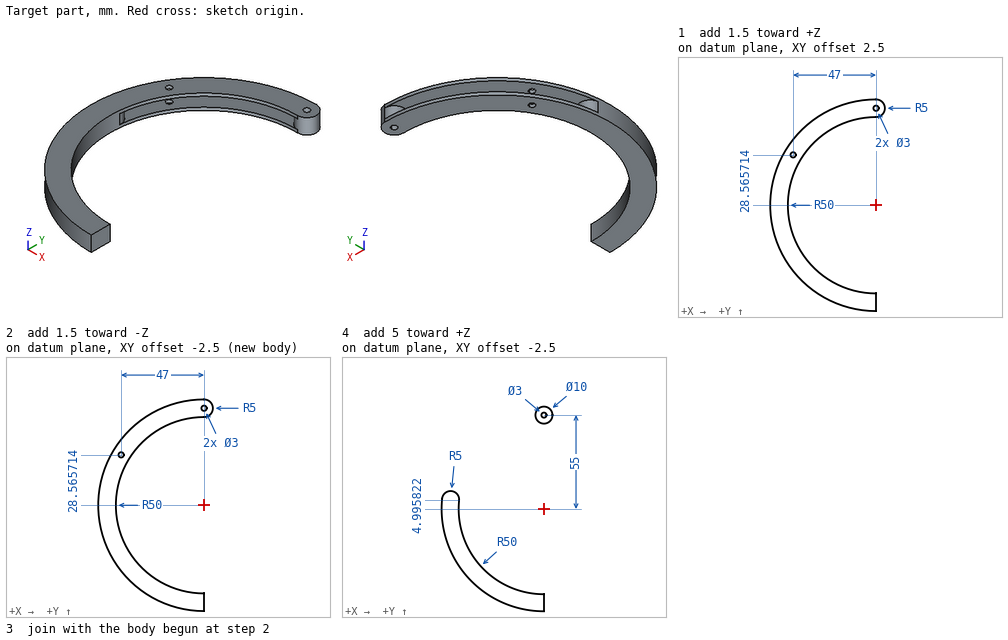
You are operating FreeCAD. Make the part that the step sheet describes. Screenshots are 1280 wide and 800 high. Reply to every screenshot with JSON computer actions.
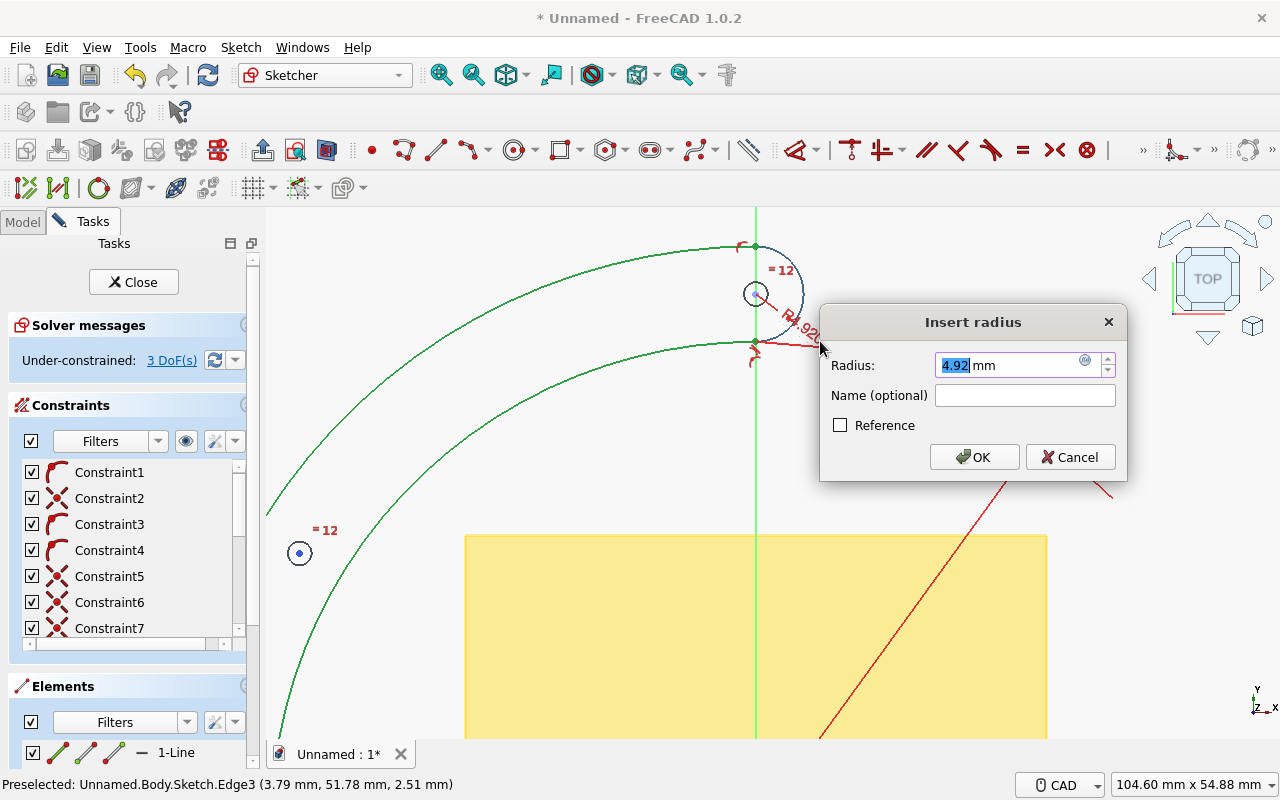
{"action": "type", "text": "5"}
{"action": "key", "text": "Return"}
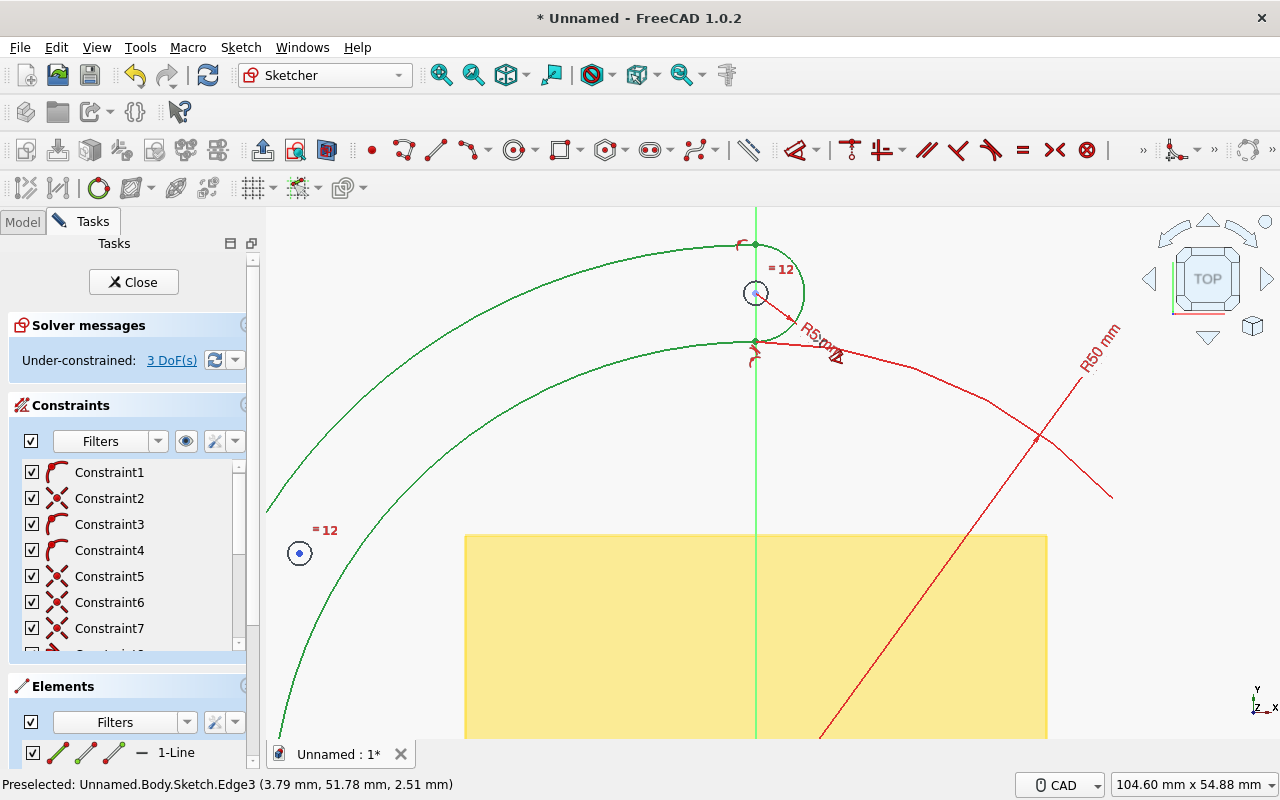
{"action": "scroll", "coordinate": [308, 545], "scroll_direction": "up", "scroll_amount": 2}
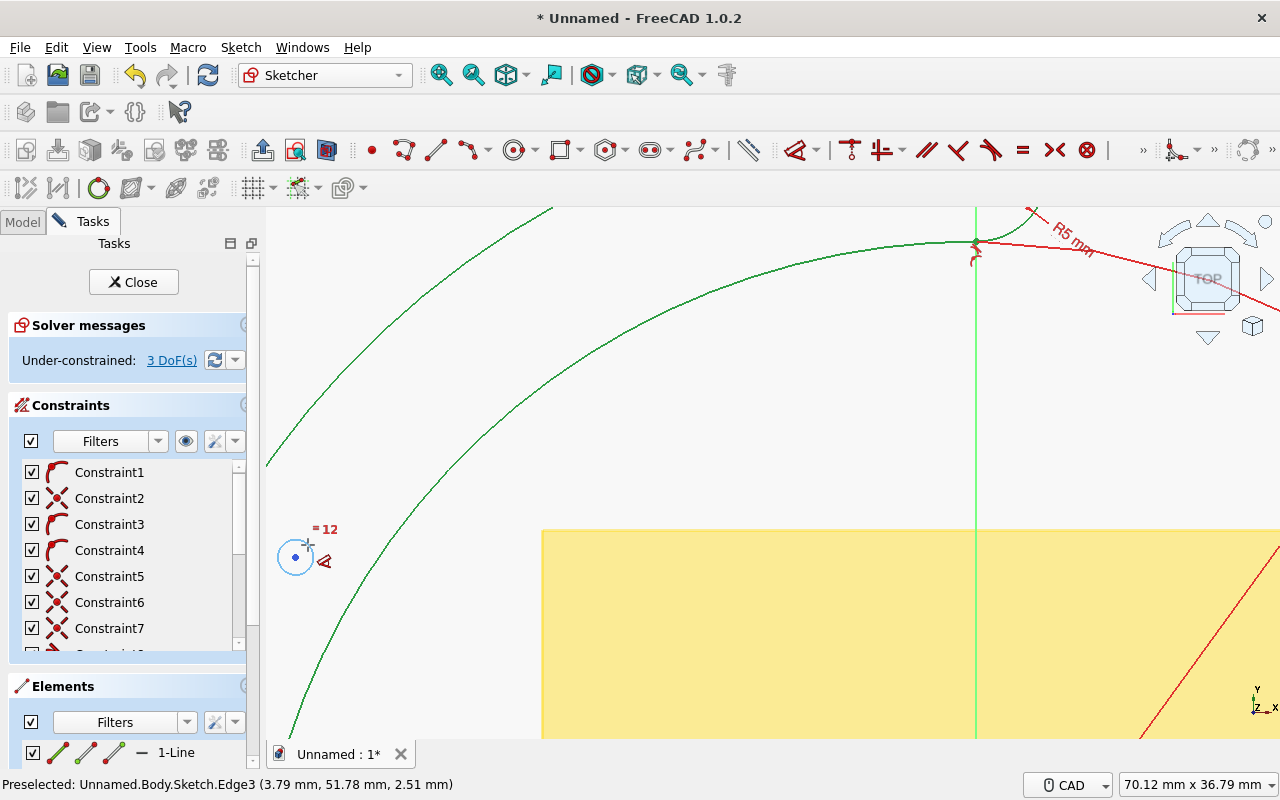
{"action": "left_click", "coordinate": [308, 545]}
{"action": "left_click", "coordinate": [331, 522]}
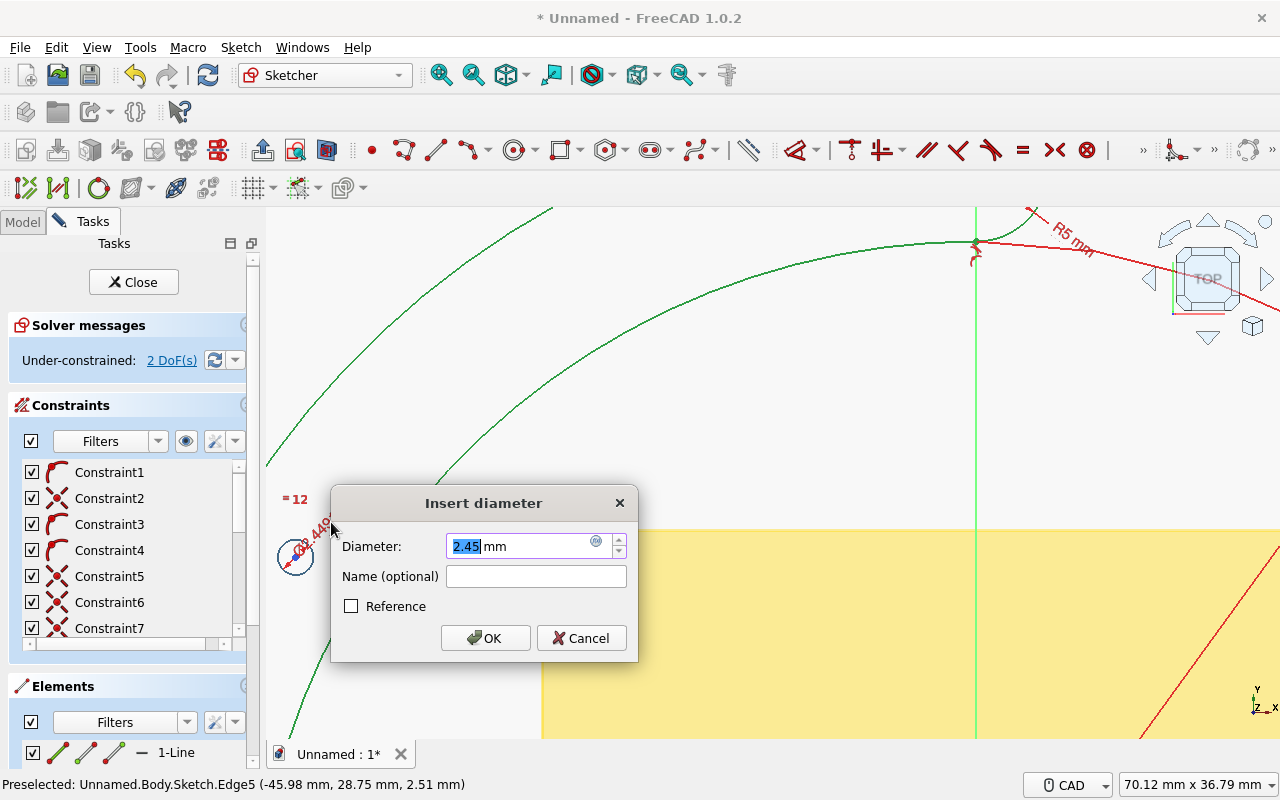
{"action": "type", "text": "3"}
{"action": "key", "text": "Return"}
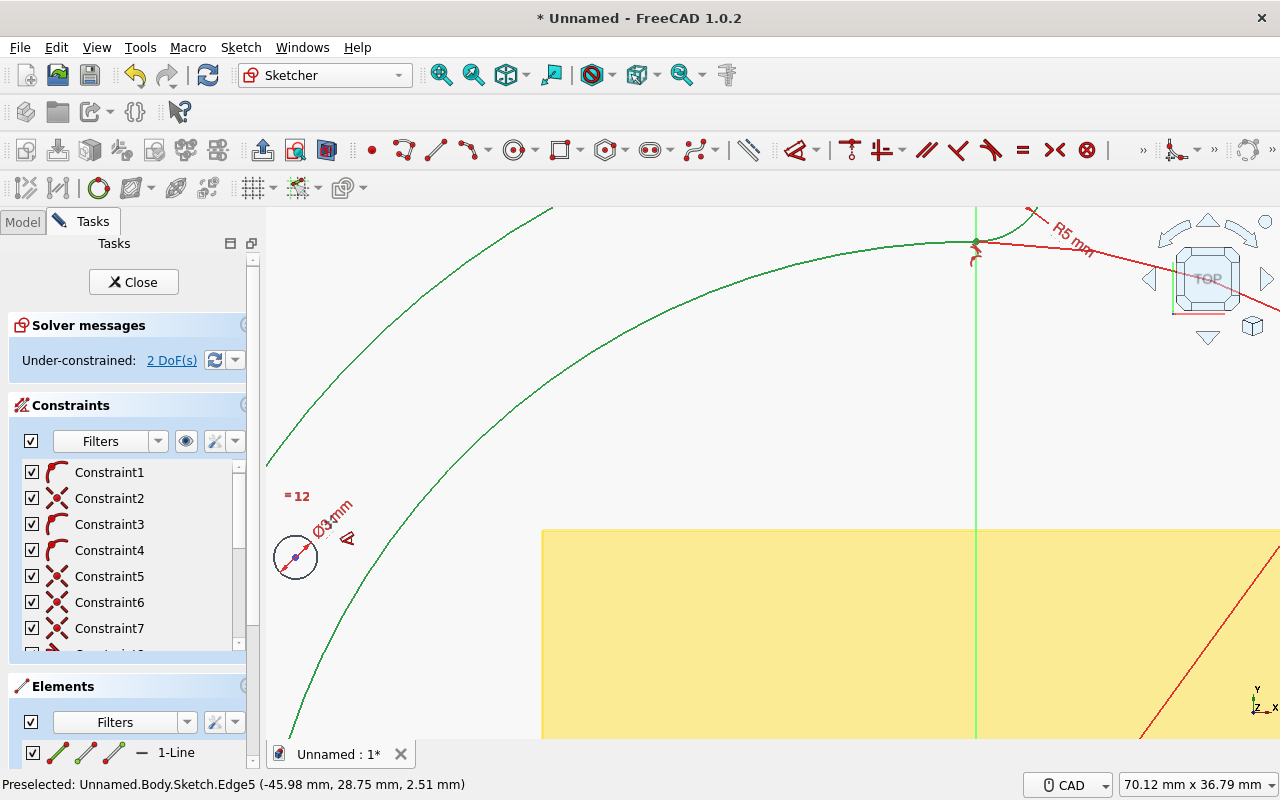
{"action": "scroll", "coordinate": [736, 349], "scroll_direction": "down", "scroll_amount": 8}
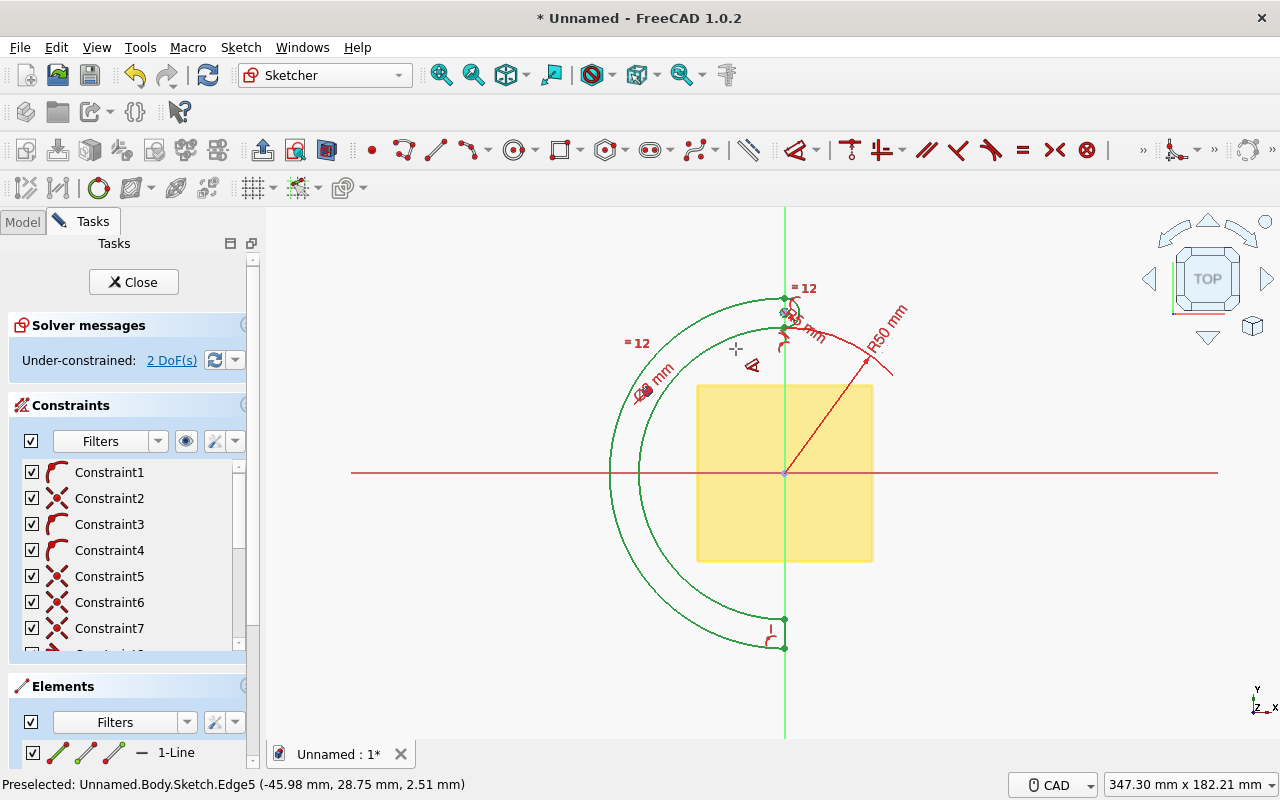
{"action": "left_click", "coordinate": [647, 391]}
{"action": "left_click", "coordinate": [748, 357]}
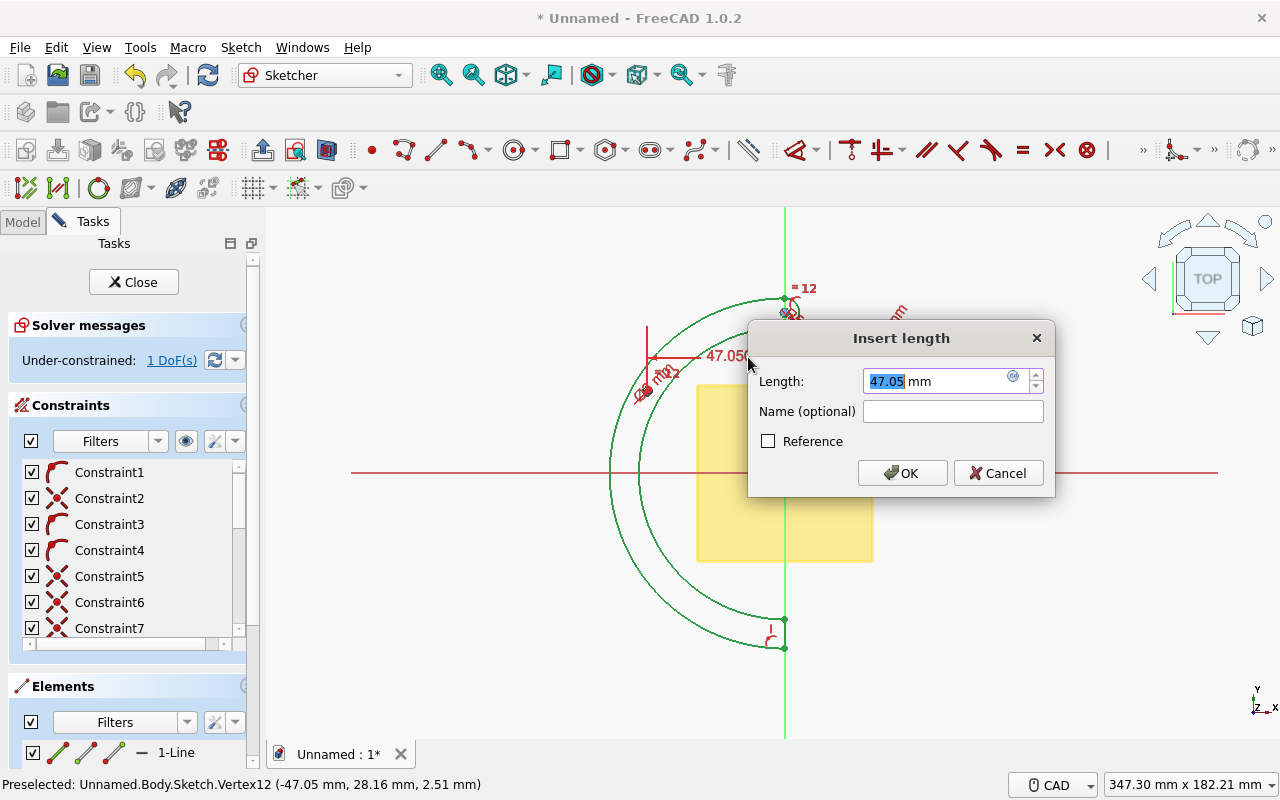
{"action": "type", "text": "47"}
{"action": "key", "text": "Return"}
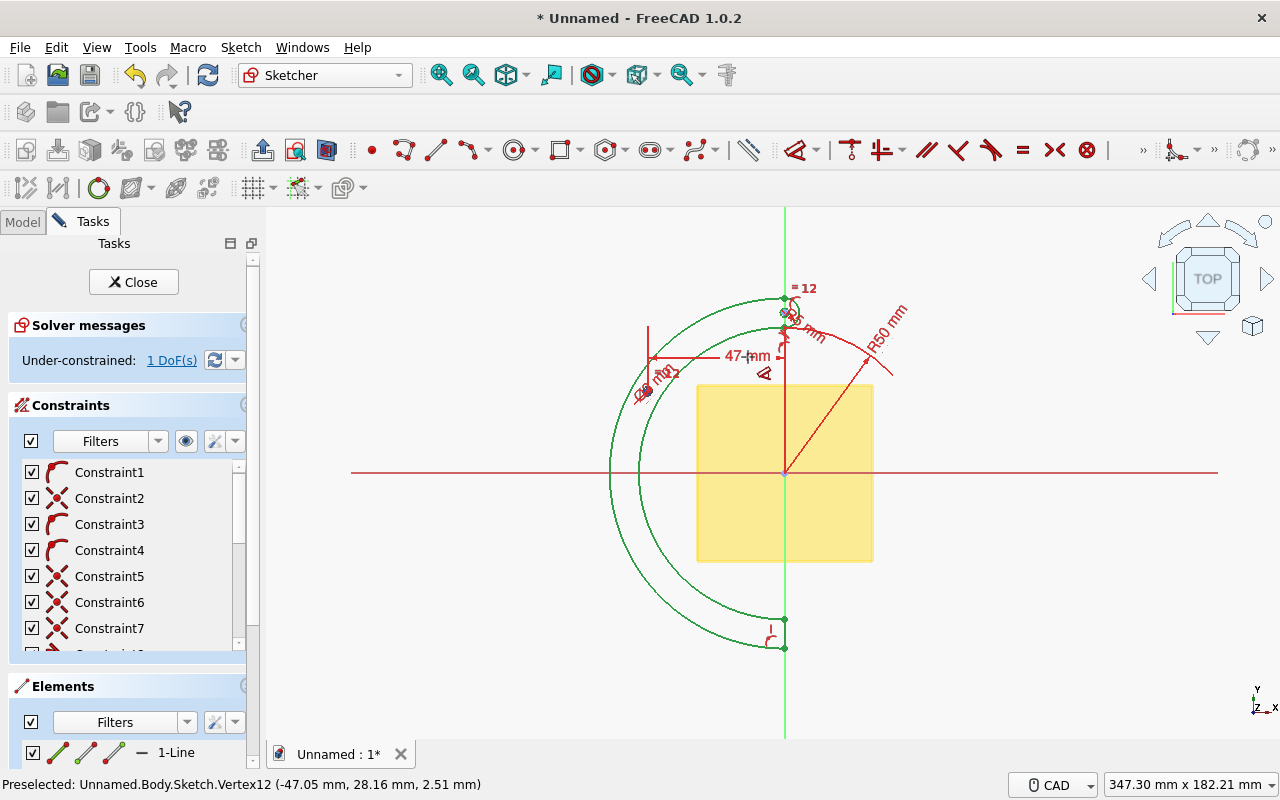
{"action": "left_click", "coordinate": [648, 391]}
{"action": "left_click", "coordinate": [819, 432]}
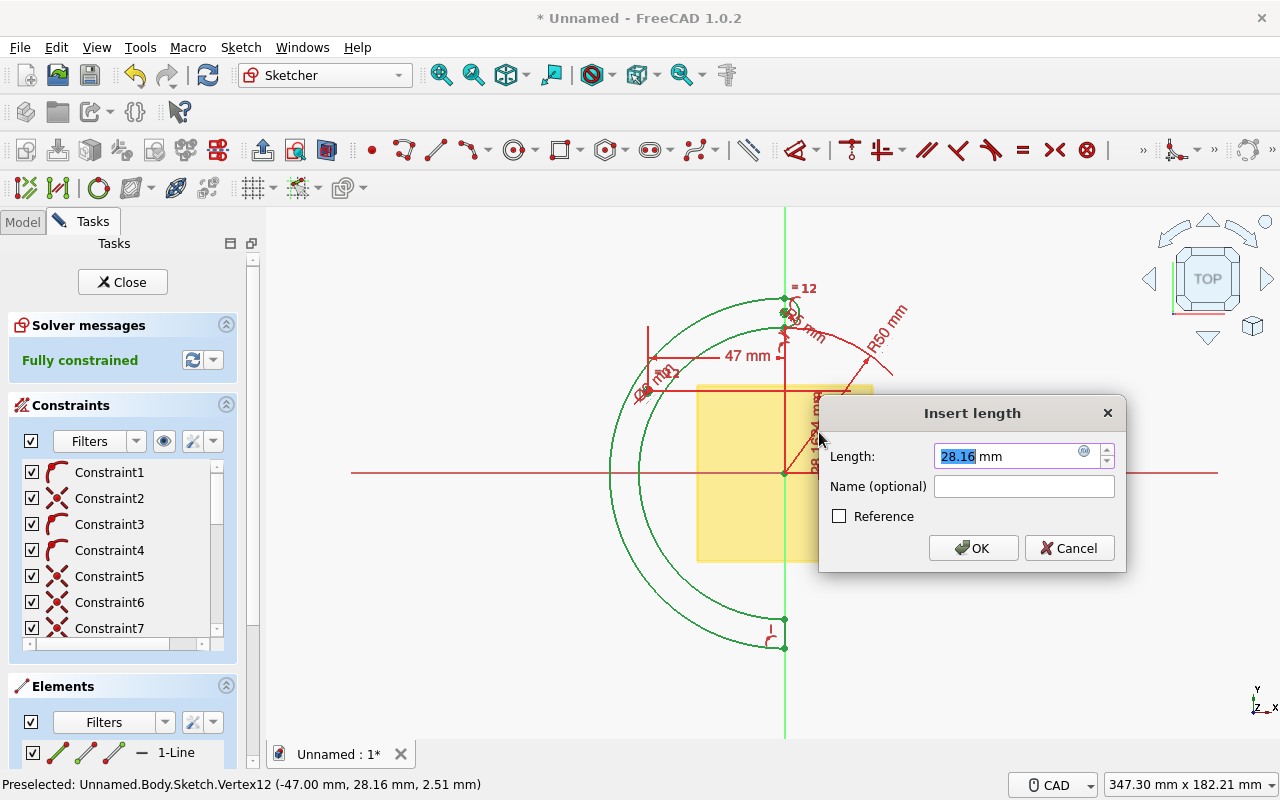
{"action": "type", "text": "28.565714"}
{"action": "key", "text": "Return"}
{"action": "key", "text": "Escape"}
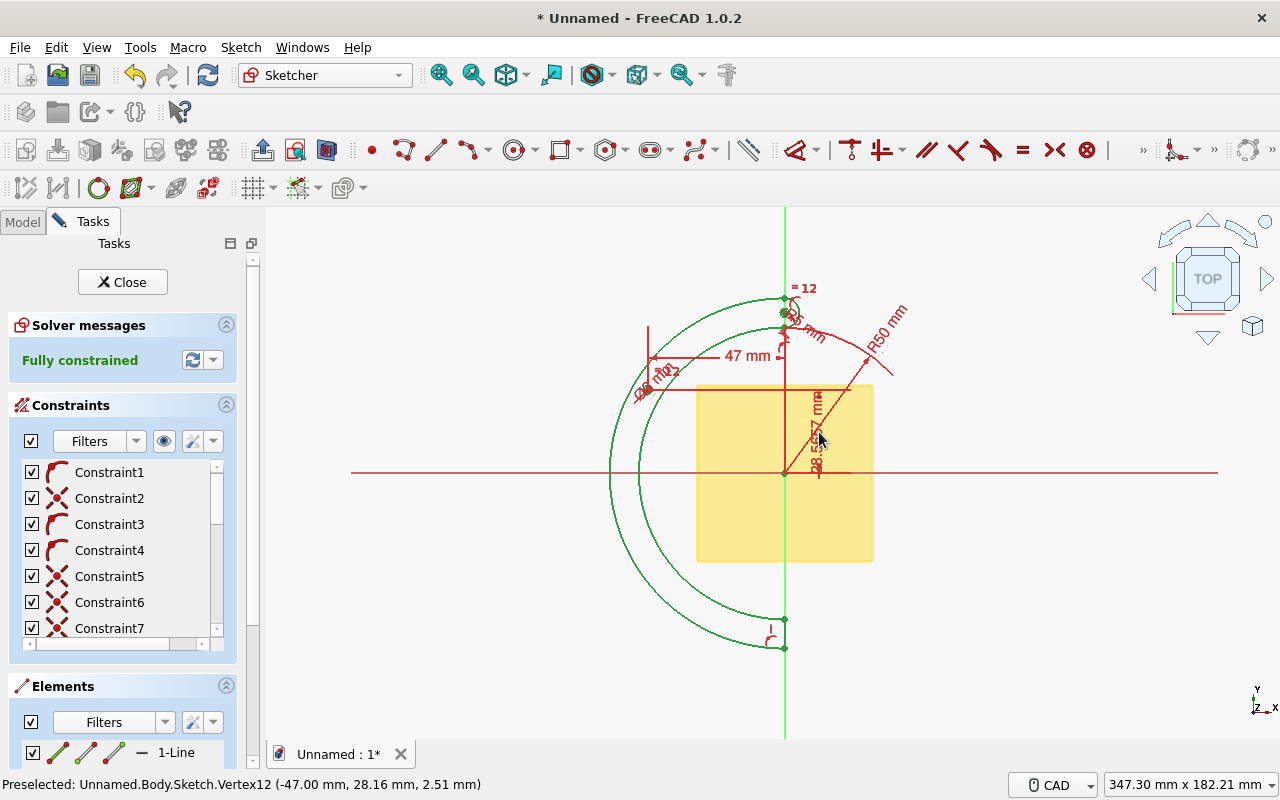
{"action": "left_click", "coordinate": [123, 282]}